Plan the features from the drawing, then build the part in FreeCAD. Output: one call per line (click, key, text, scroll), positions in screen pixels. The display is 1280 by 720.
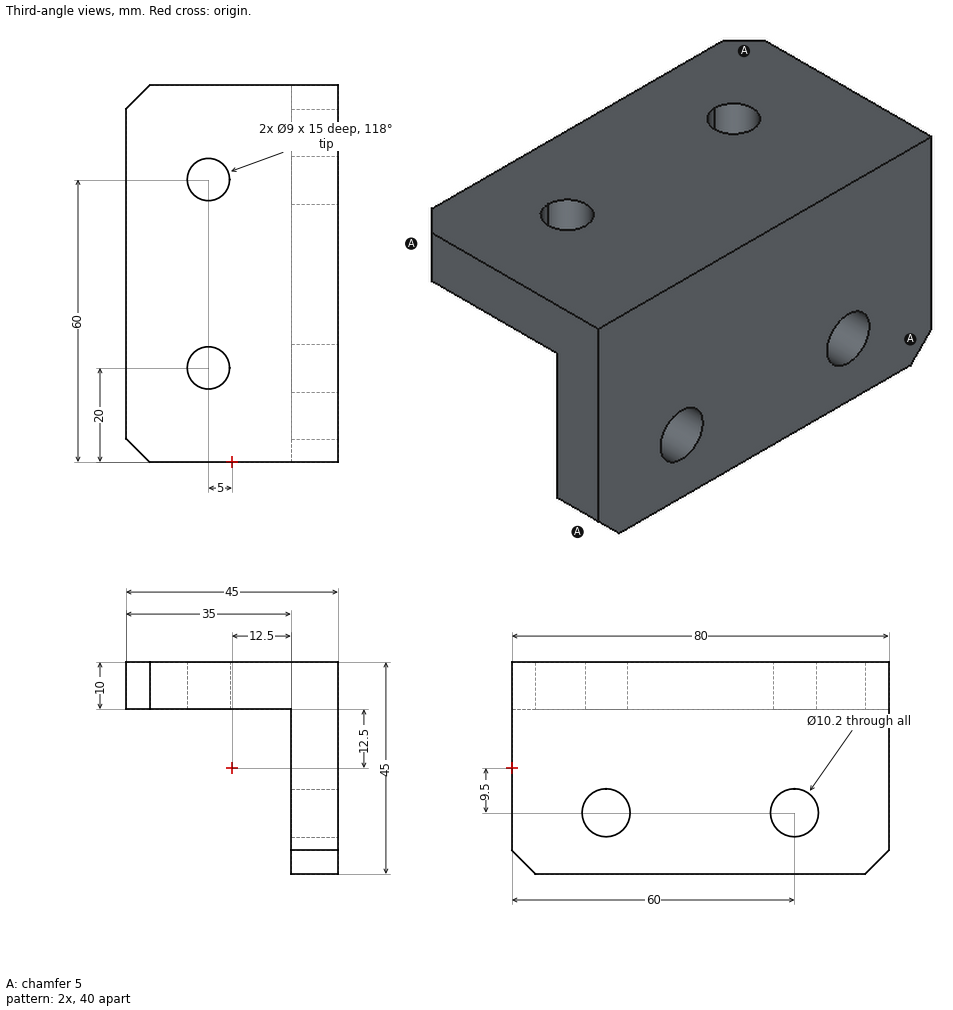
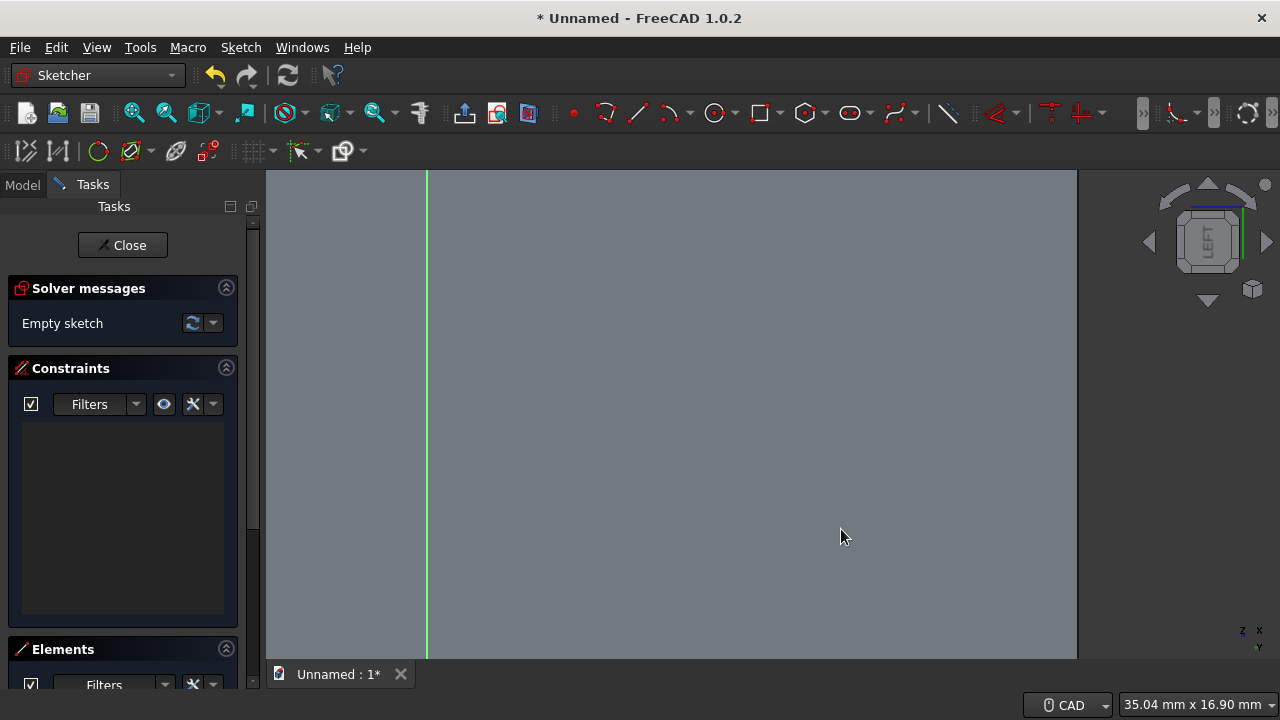
click(716, 114)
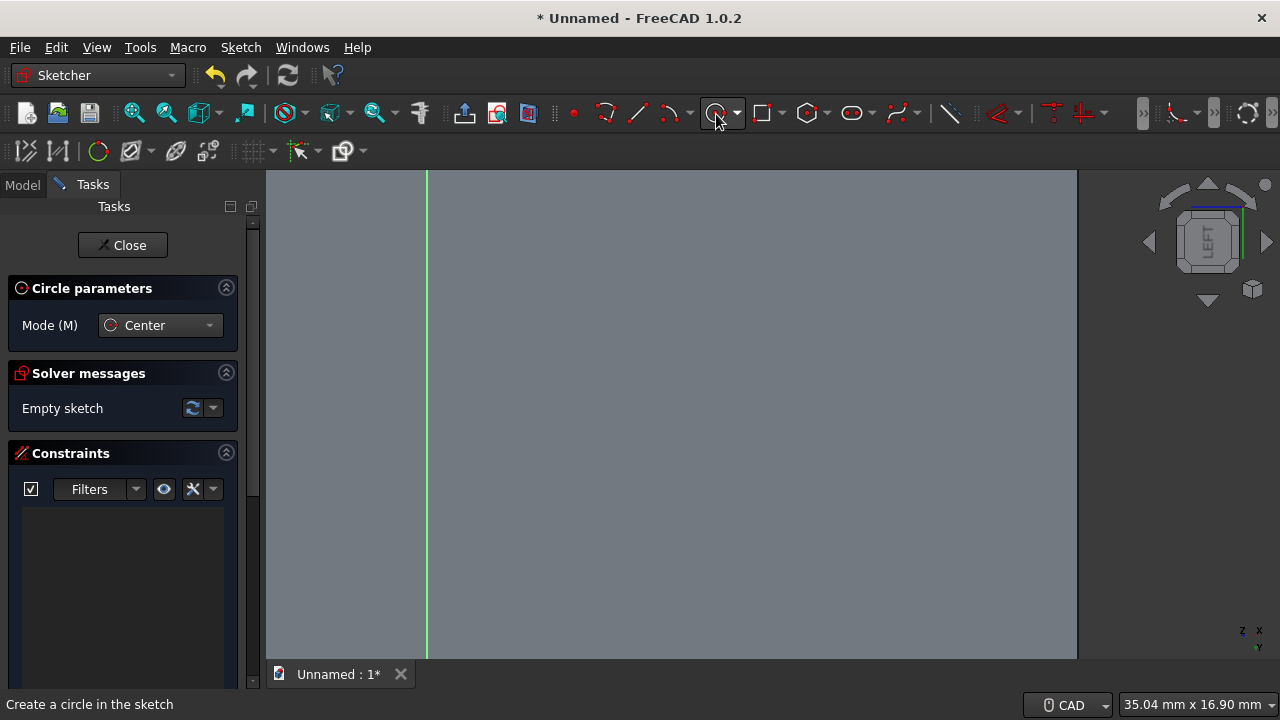
click(702, 411)
move(806, 307)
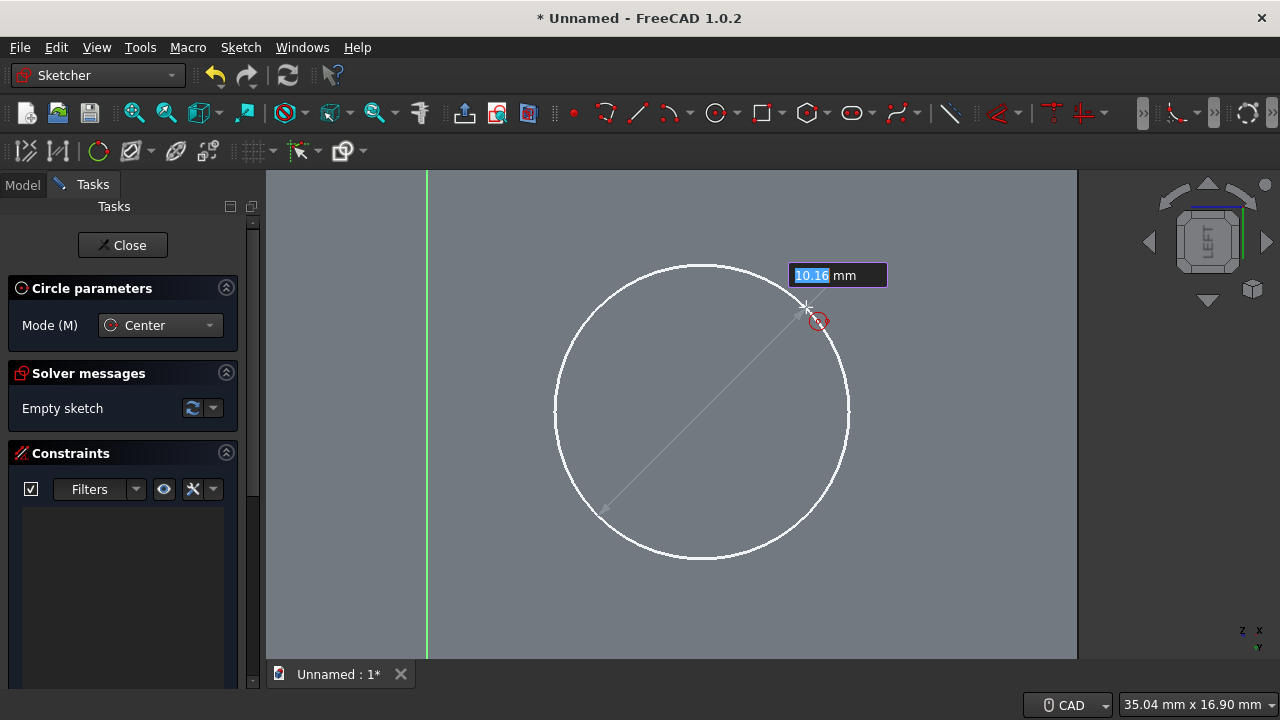
text(10.2)
key(Return)
key(Escape)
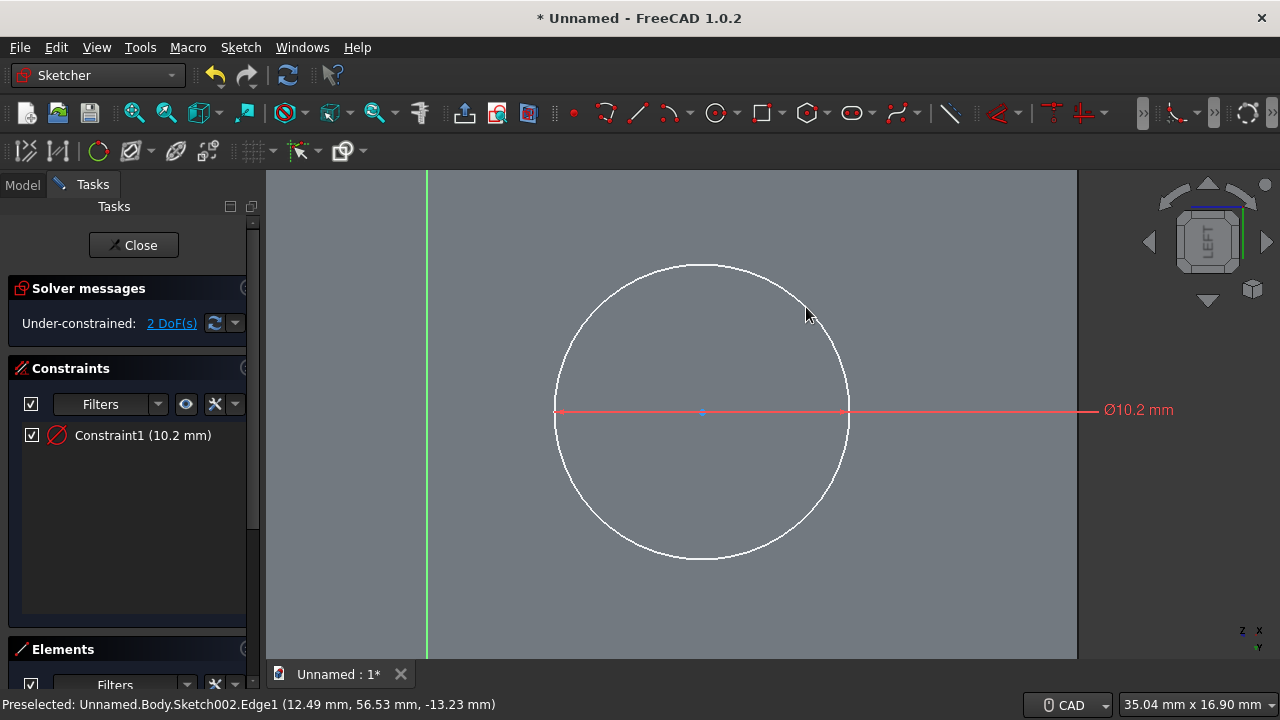
key(d)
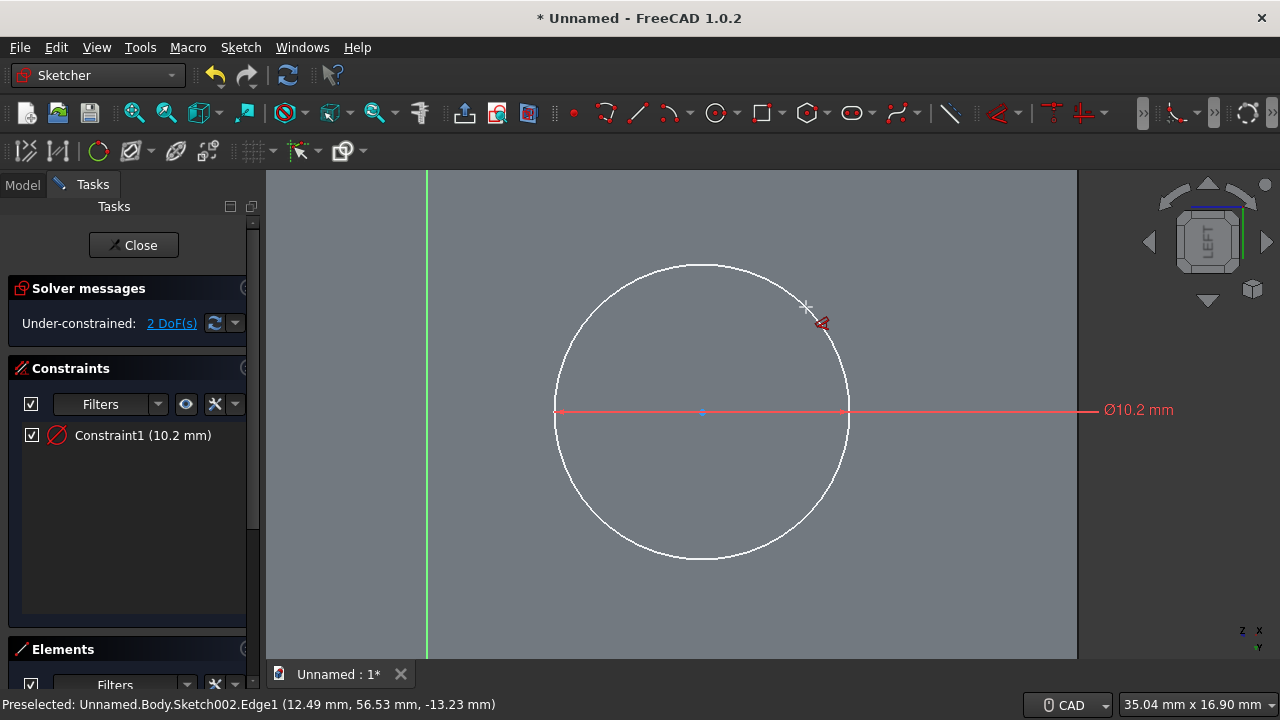
click(702, 412)
click(393, 305)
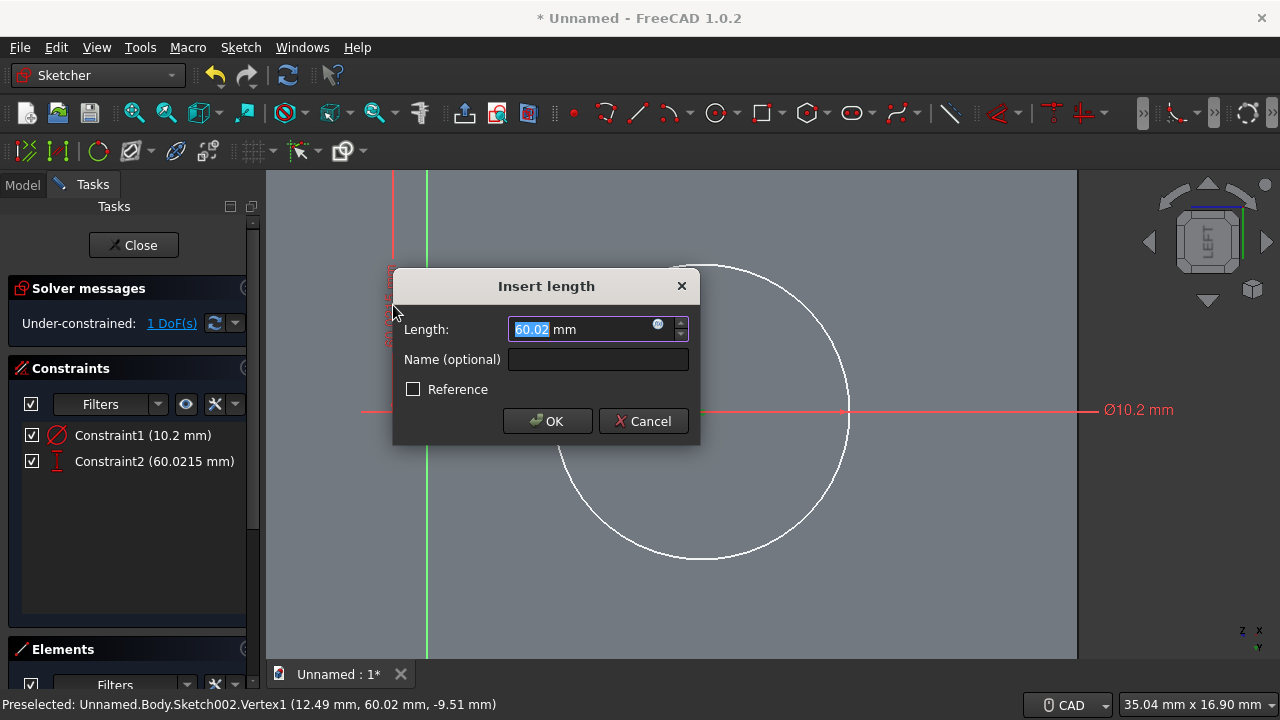
text(60)
key(Return)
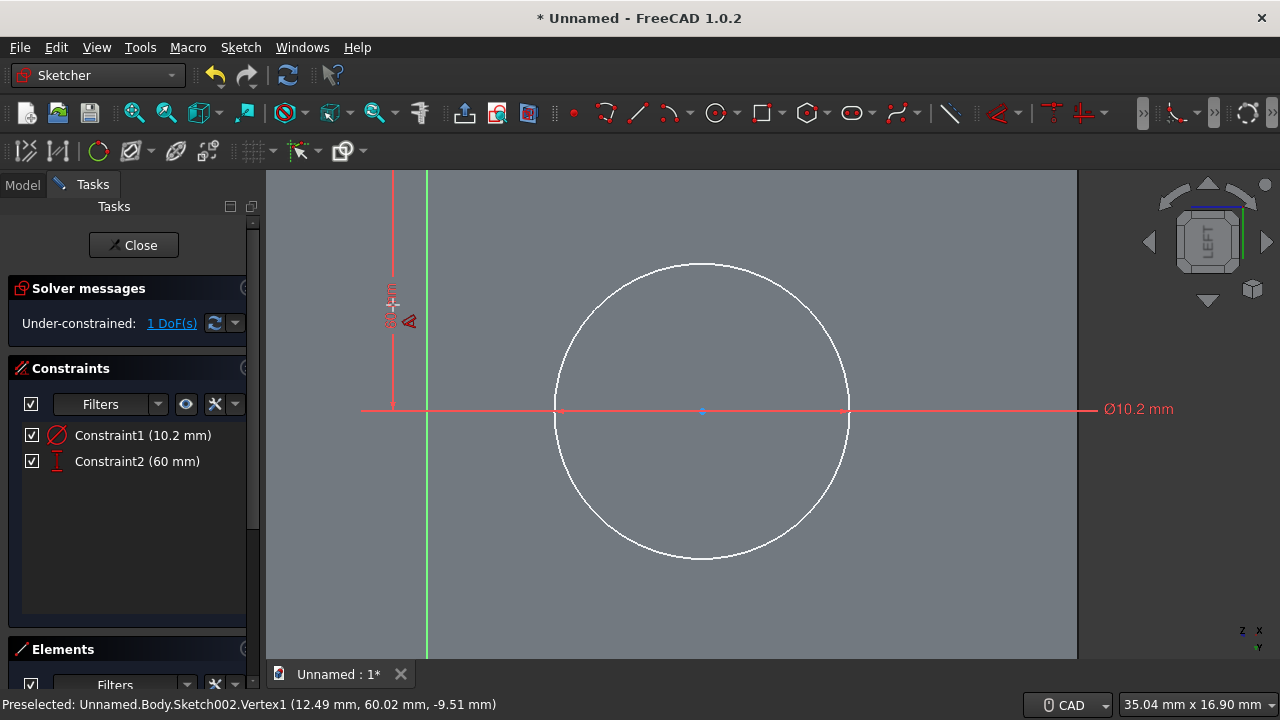
click(702, 411)
click(501, 445)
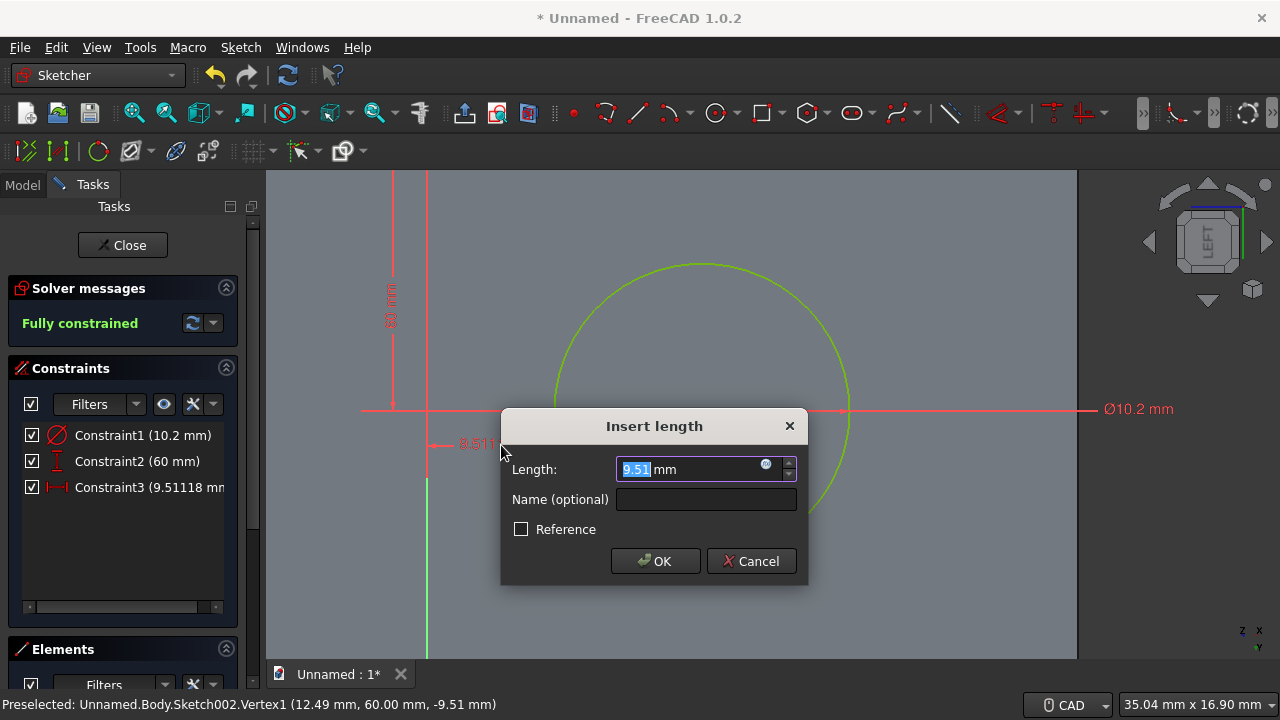
text(9.5)
key(Return)
key(Escape)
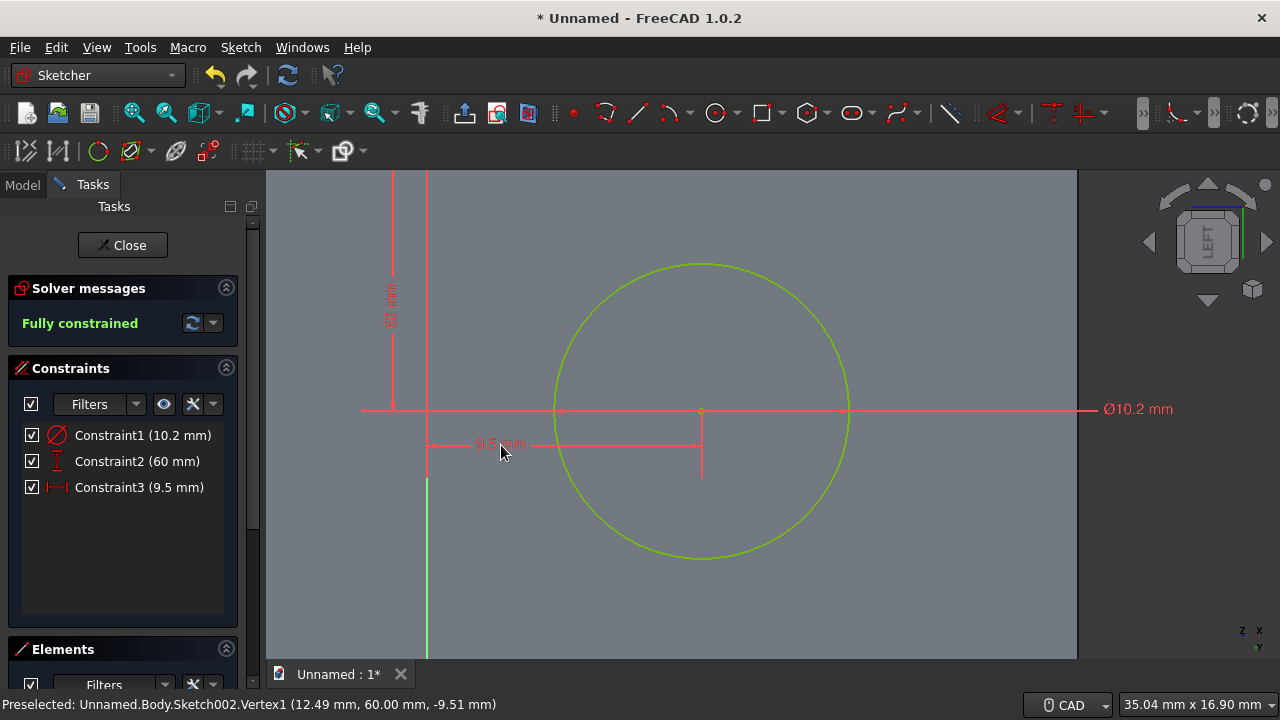
click(123, 245)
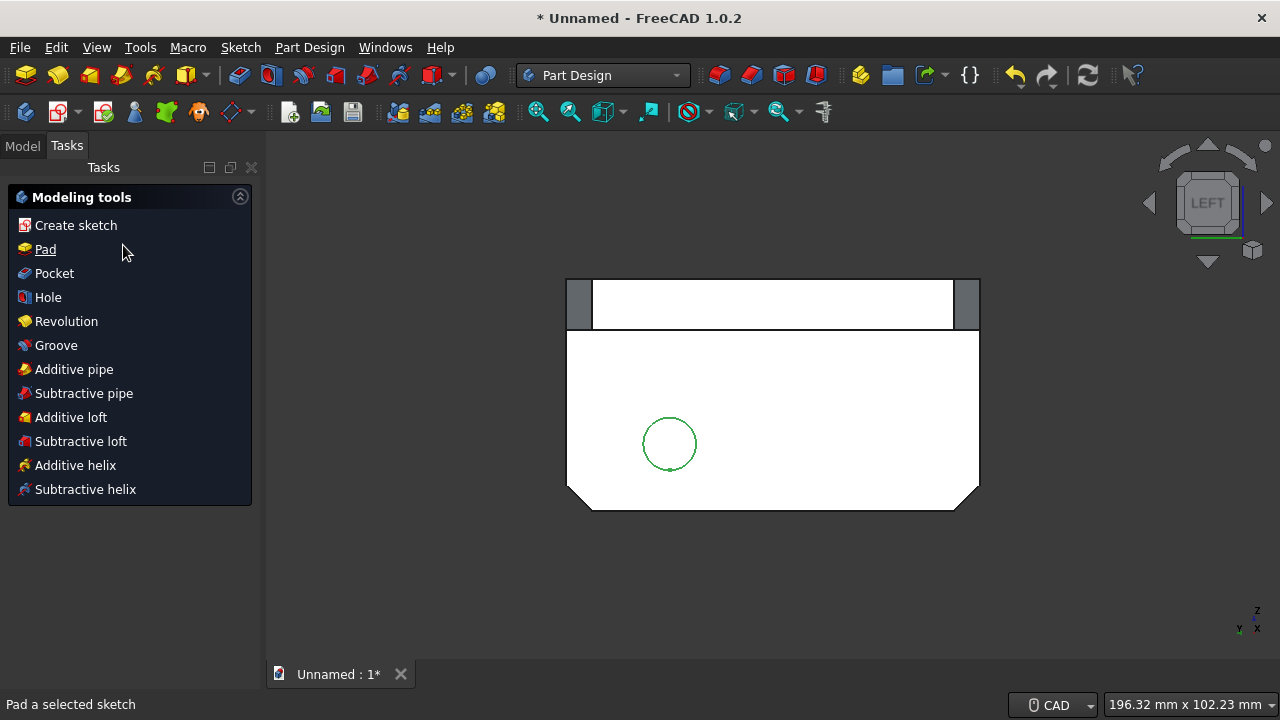
click(272, 76)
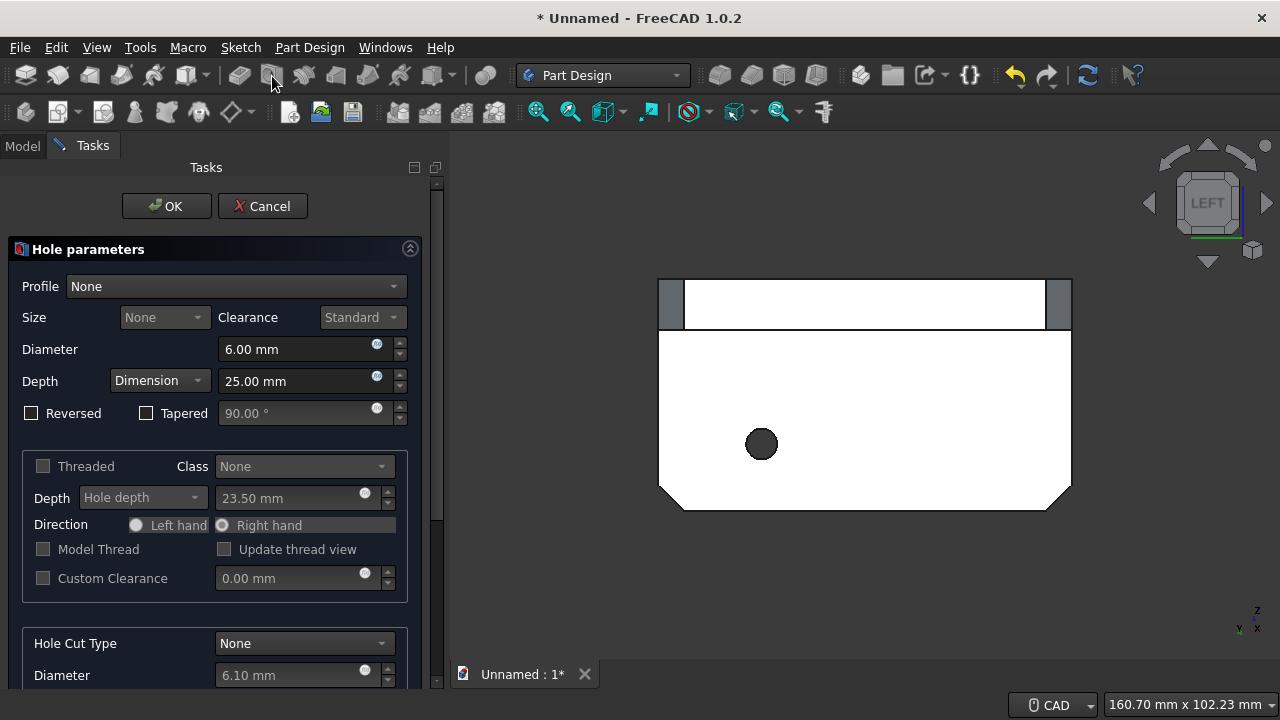
triple_click(305, 349)